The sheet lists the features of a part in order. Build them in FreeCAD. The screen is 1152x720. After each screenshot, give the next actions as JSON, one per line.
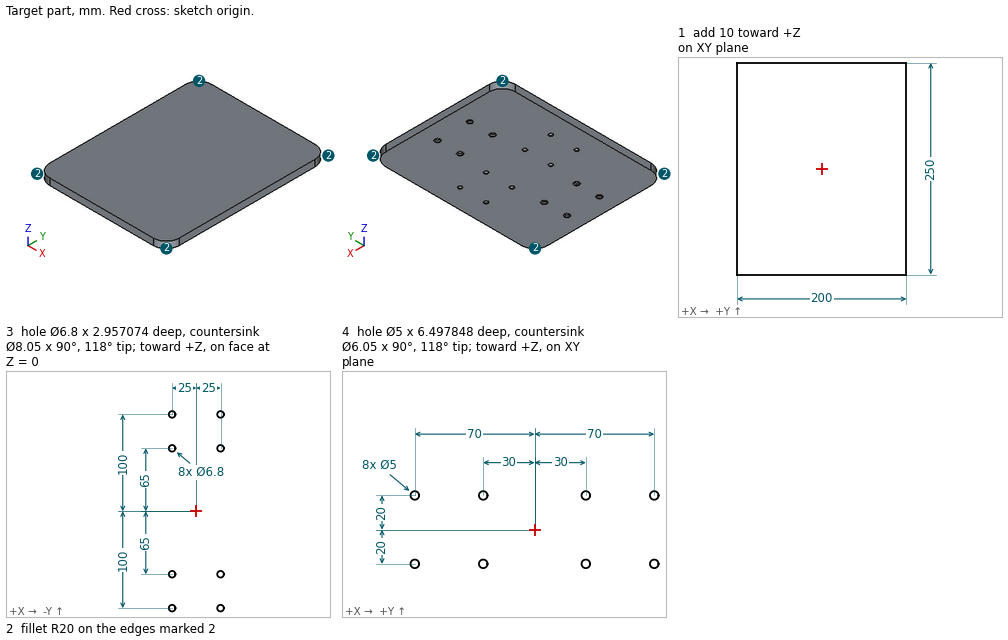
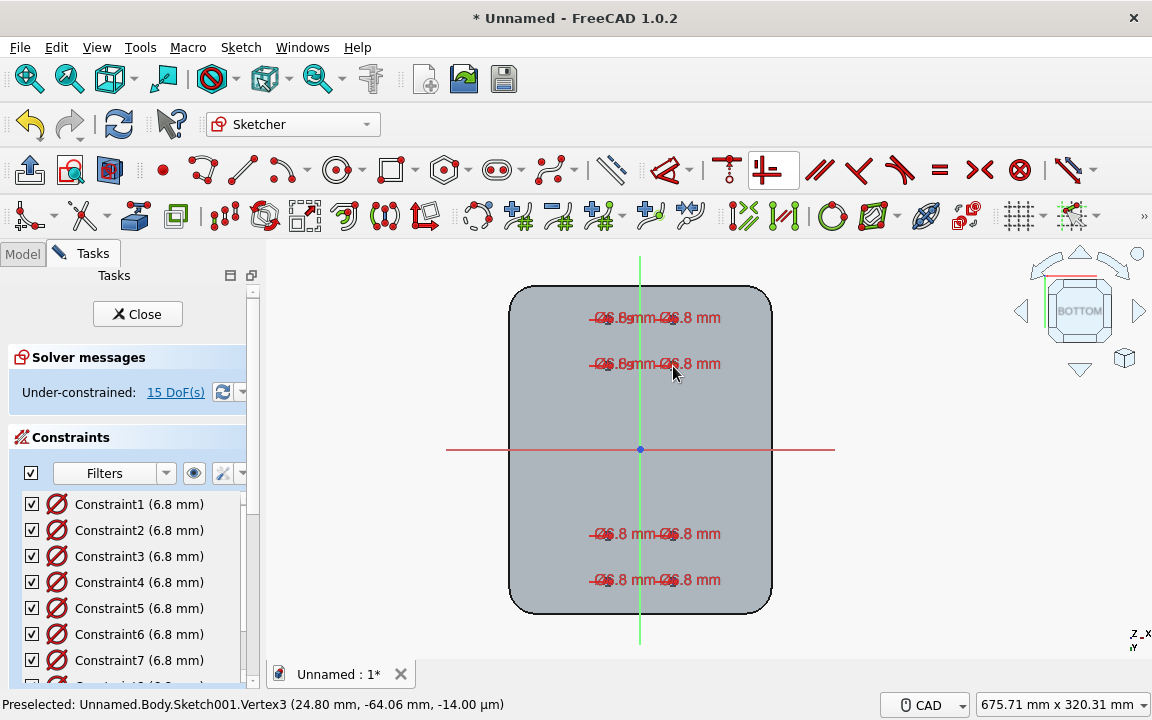
{"action": "key", "text": "h"}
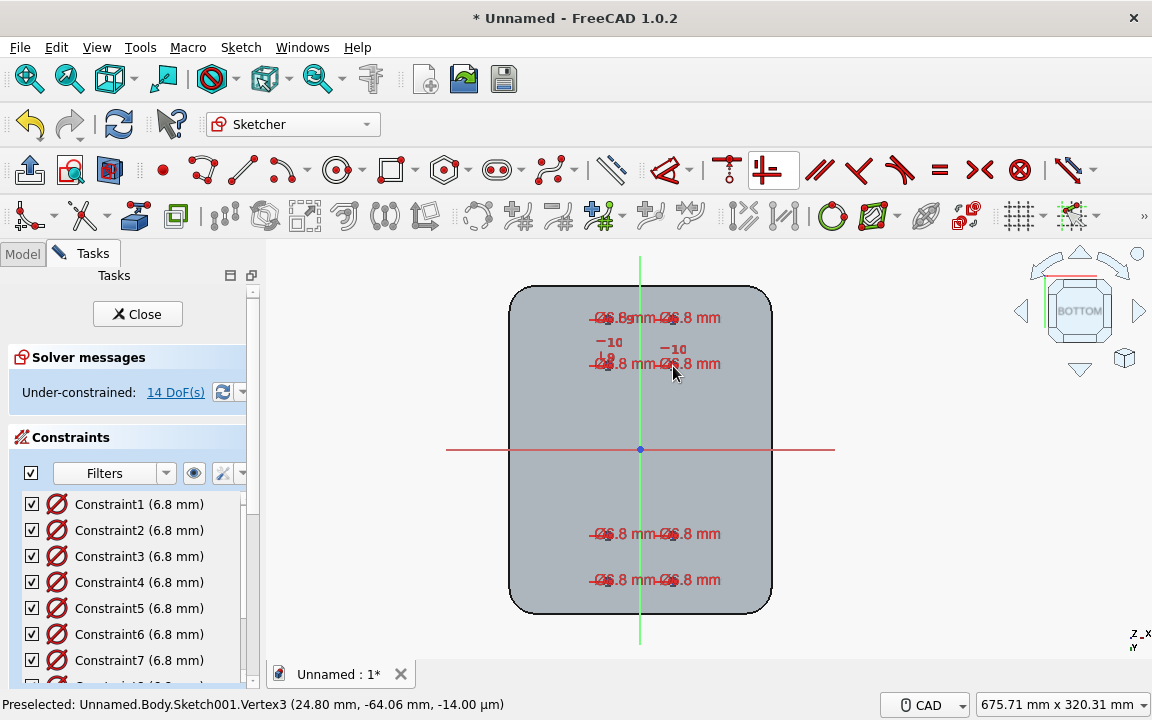
{"action": "left_click", "coordinate": [673, 366]}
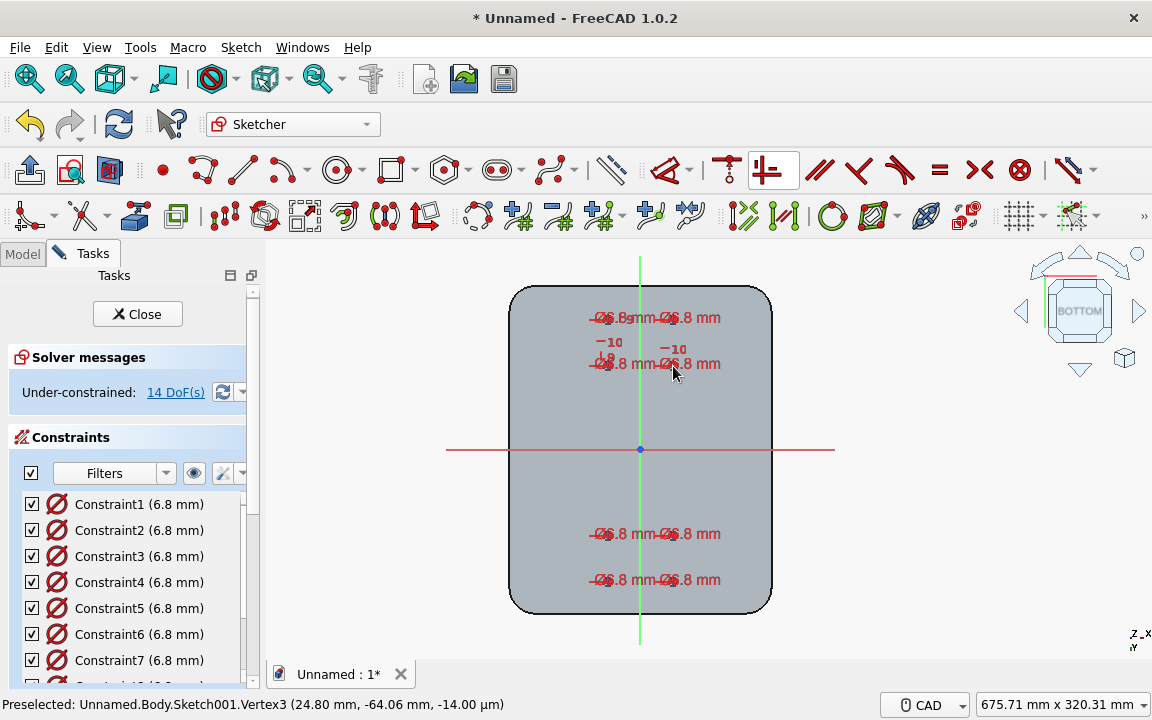
{"action": "left_click", "coordinate": [673, 320]}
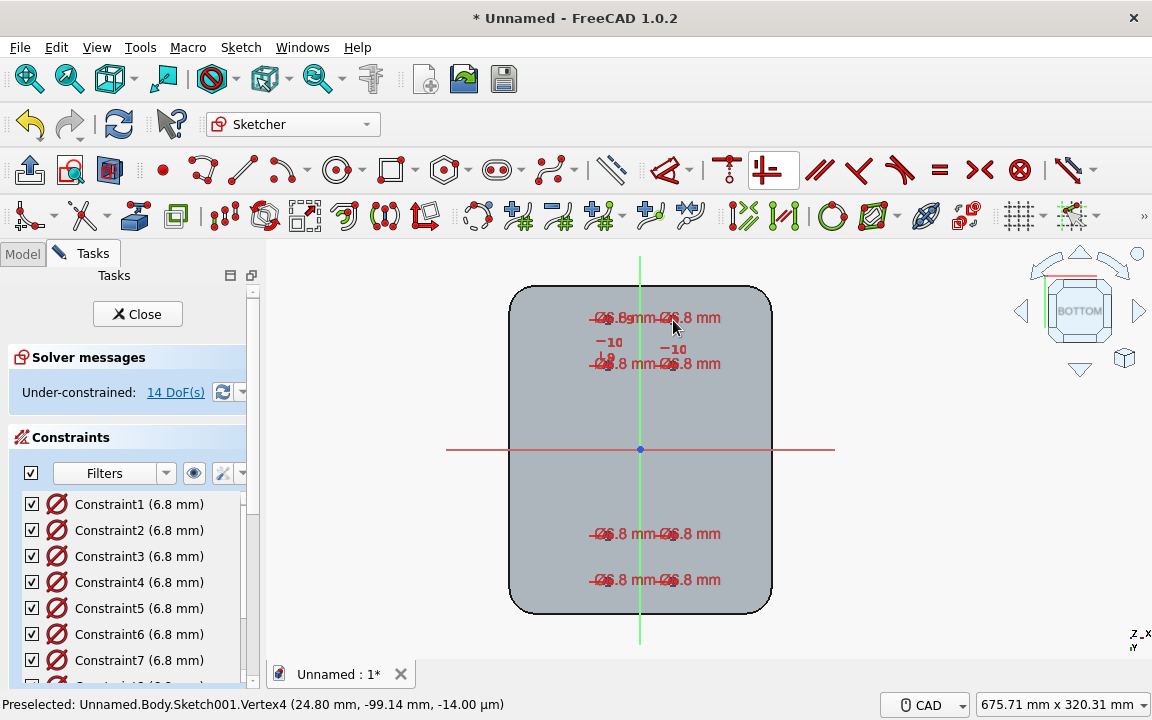
{"action": "key", "text": "v"}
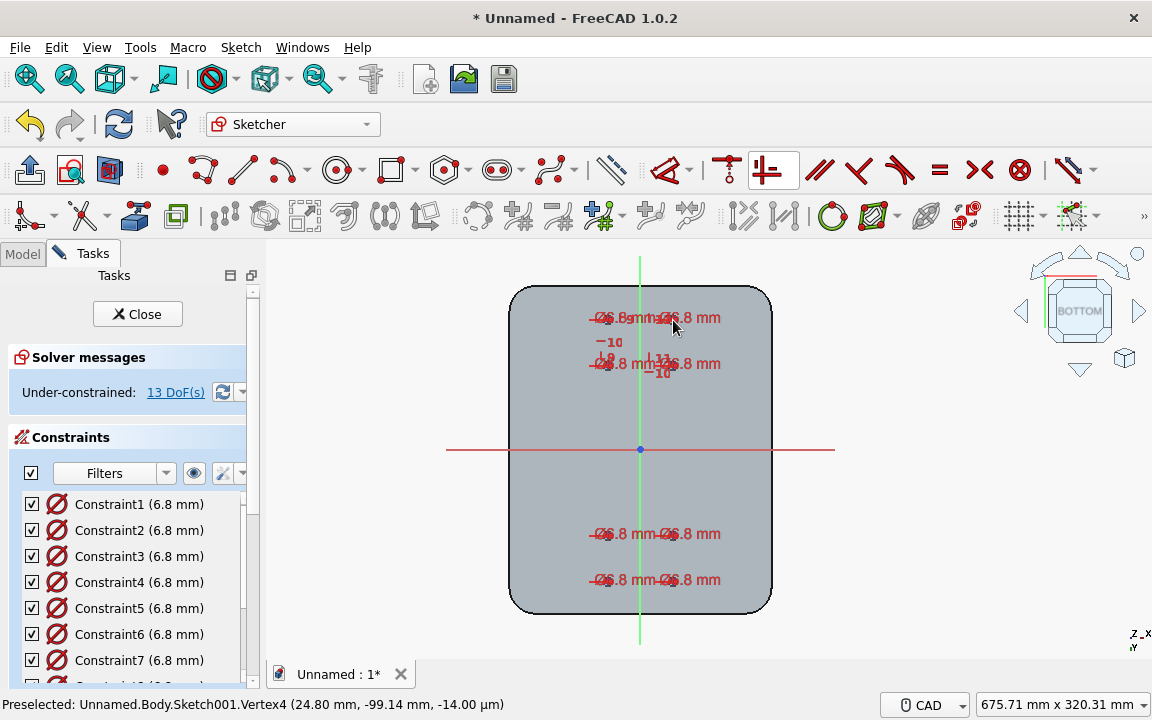
{"action": "left_click", "coordinate": [608, 320]}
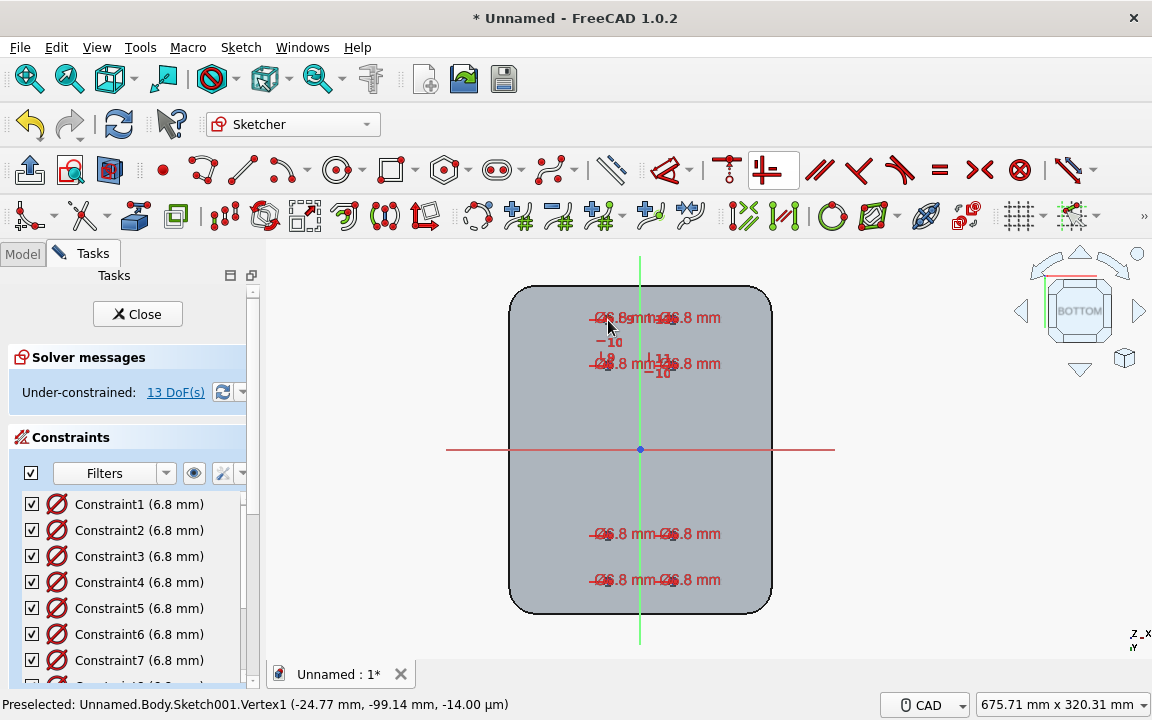
{"action": "left_click", "coordinate": [673, 320]}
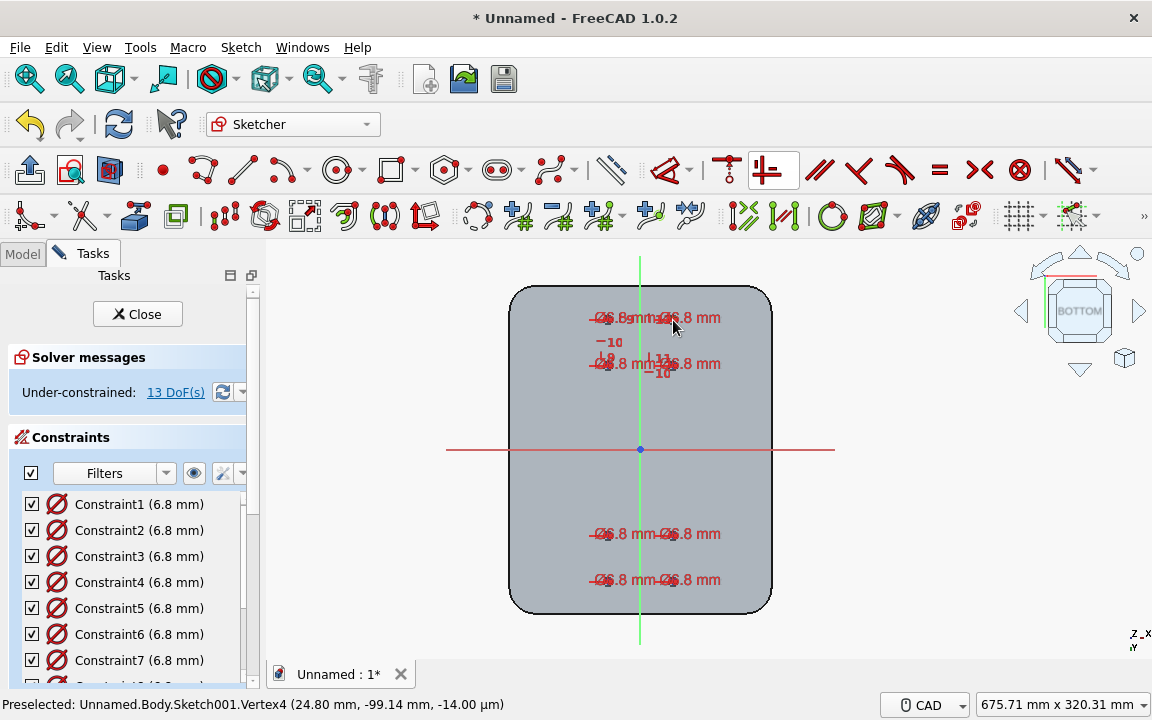
{"action": "key", "text": "h"}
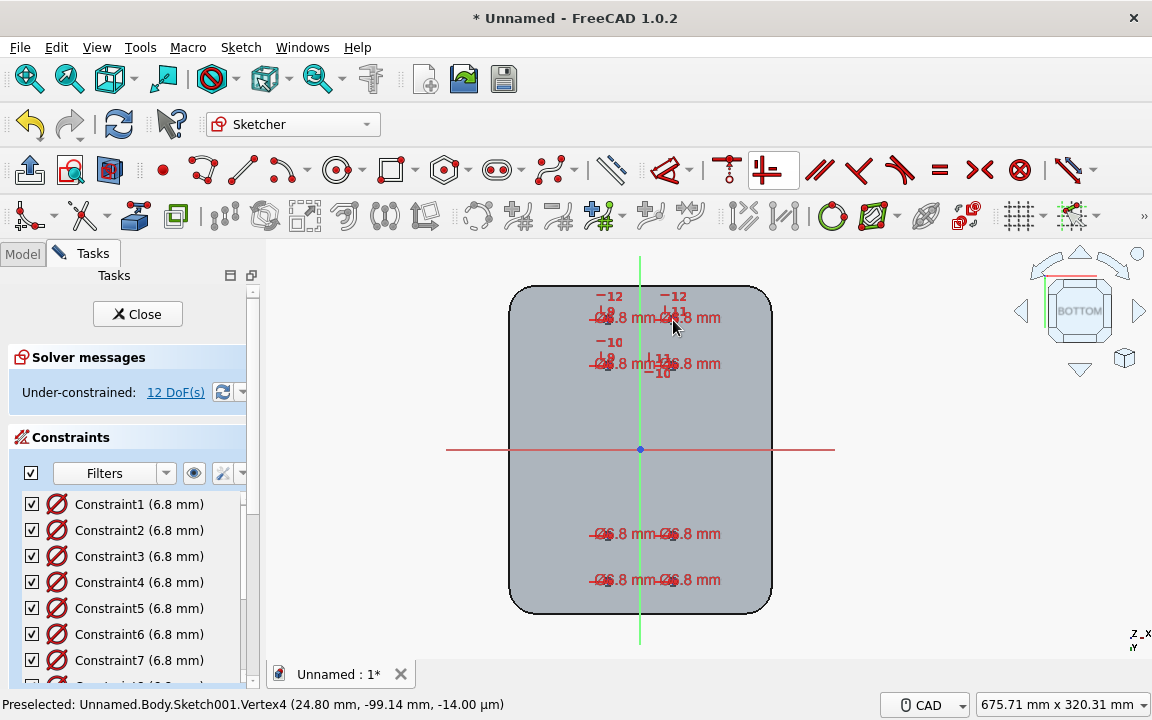
{"action": "left_click", "coordinate": [608, 366]}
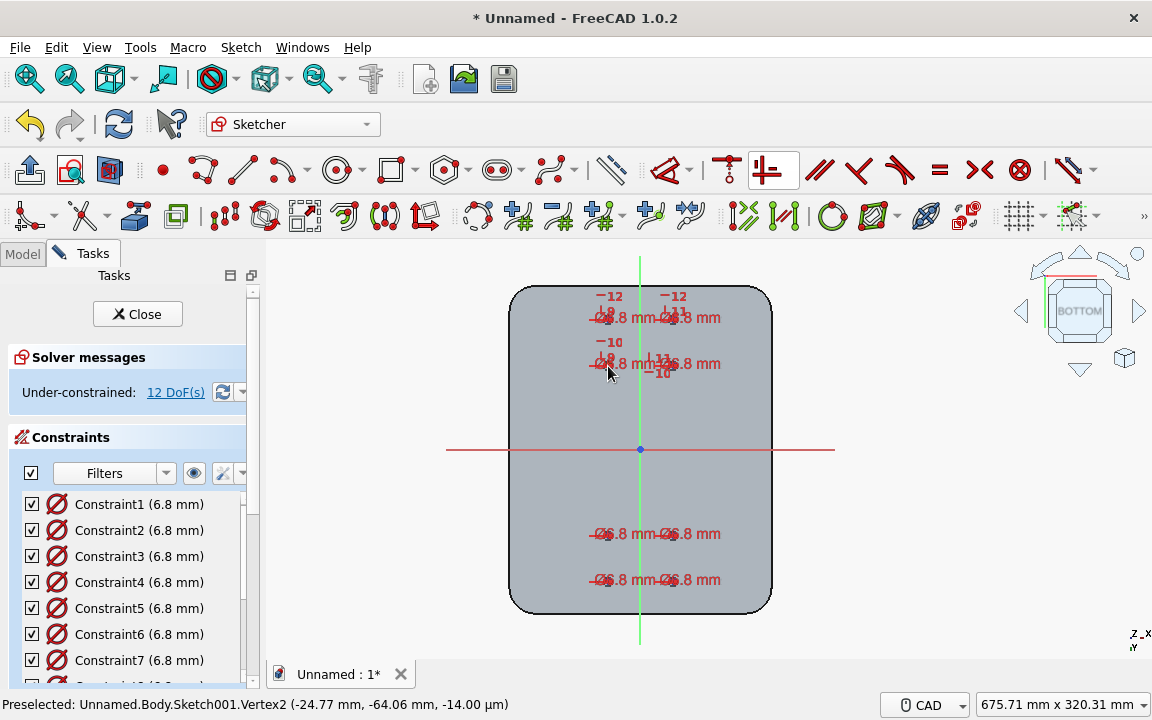
{"action": "left_click", "coordinate": [608, 582]}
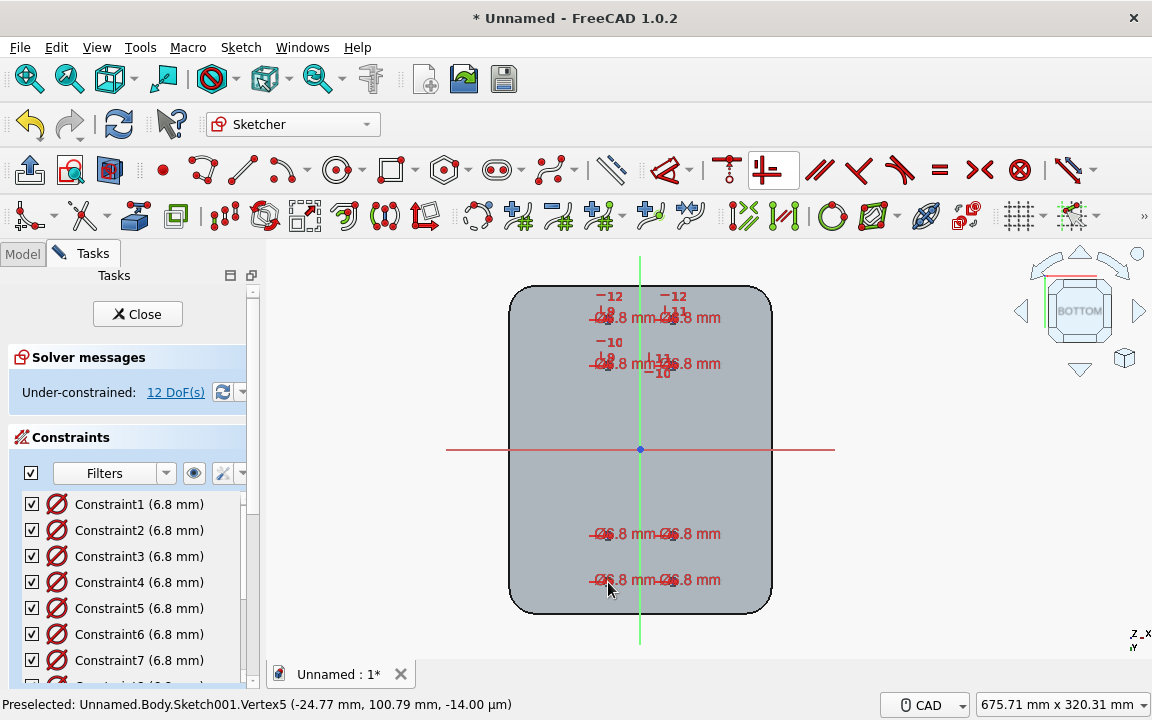
{"action": "key", "text": "v"}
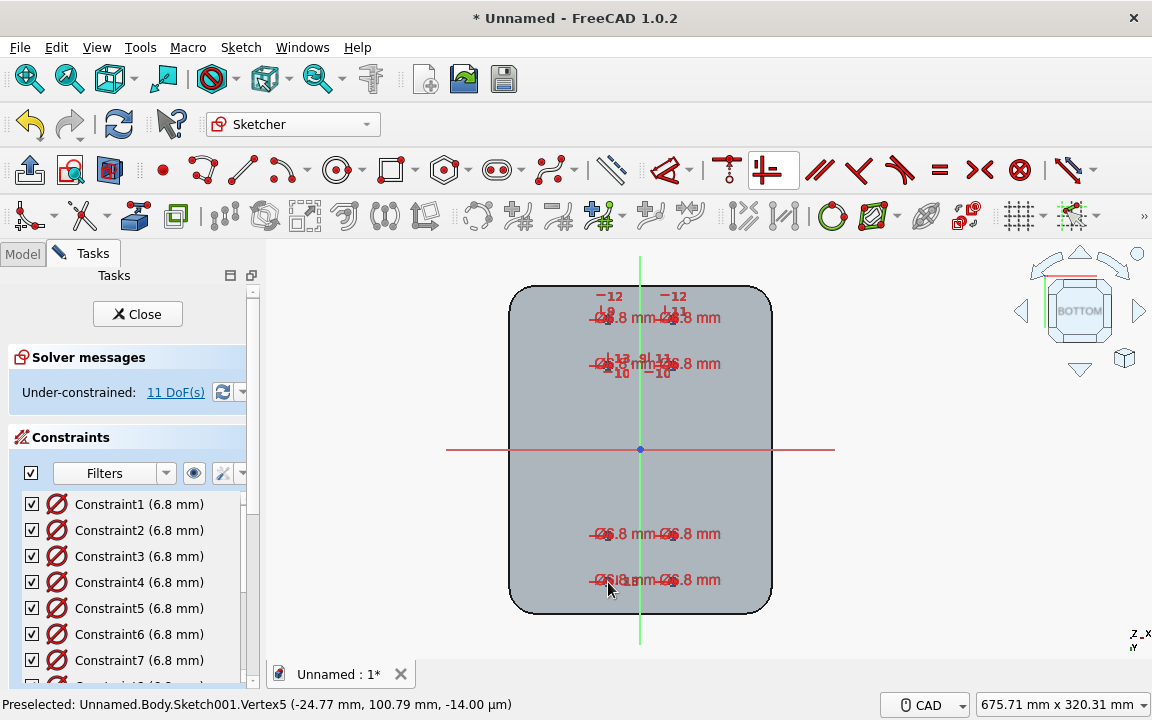
{"action": "left_click", "coordinate": [608, 582]}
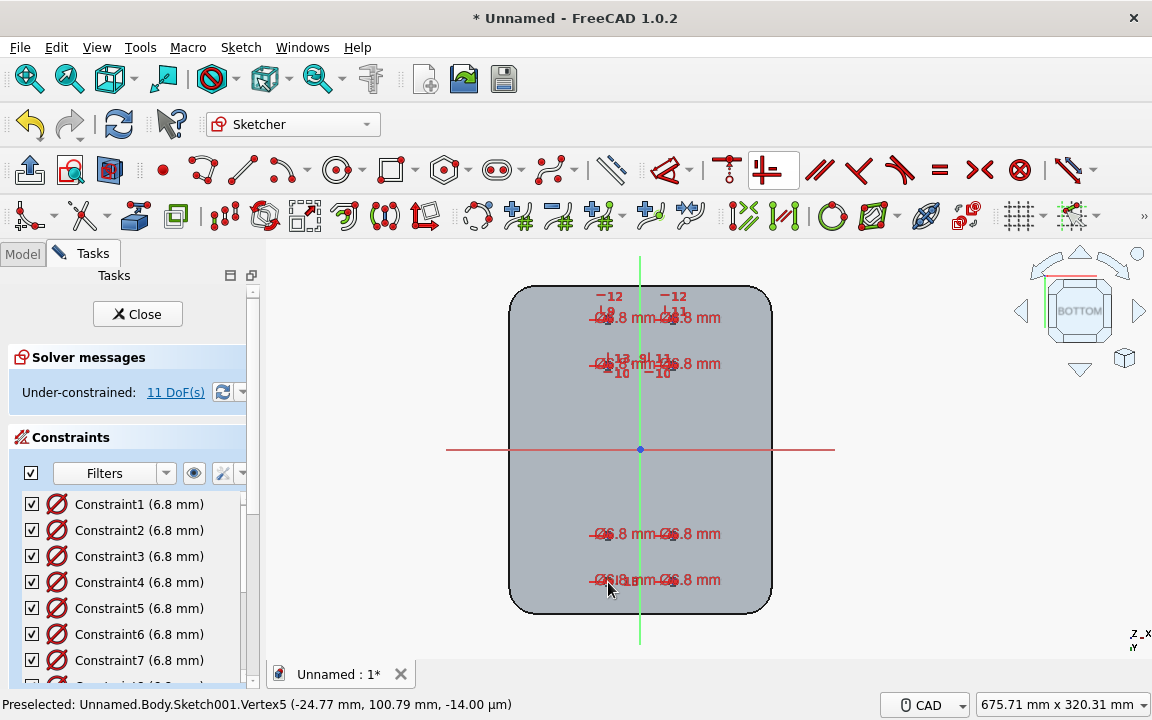
{"action": "left_click", "coordinate": [608, 536]}